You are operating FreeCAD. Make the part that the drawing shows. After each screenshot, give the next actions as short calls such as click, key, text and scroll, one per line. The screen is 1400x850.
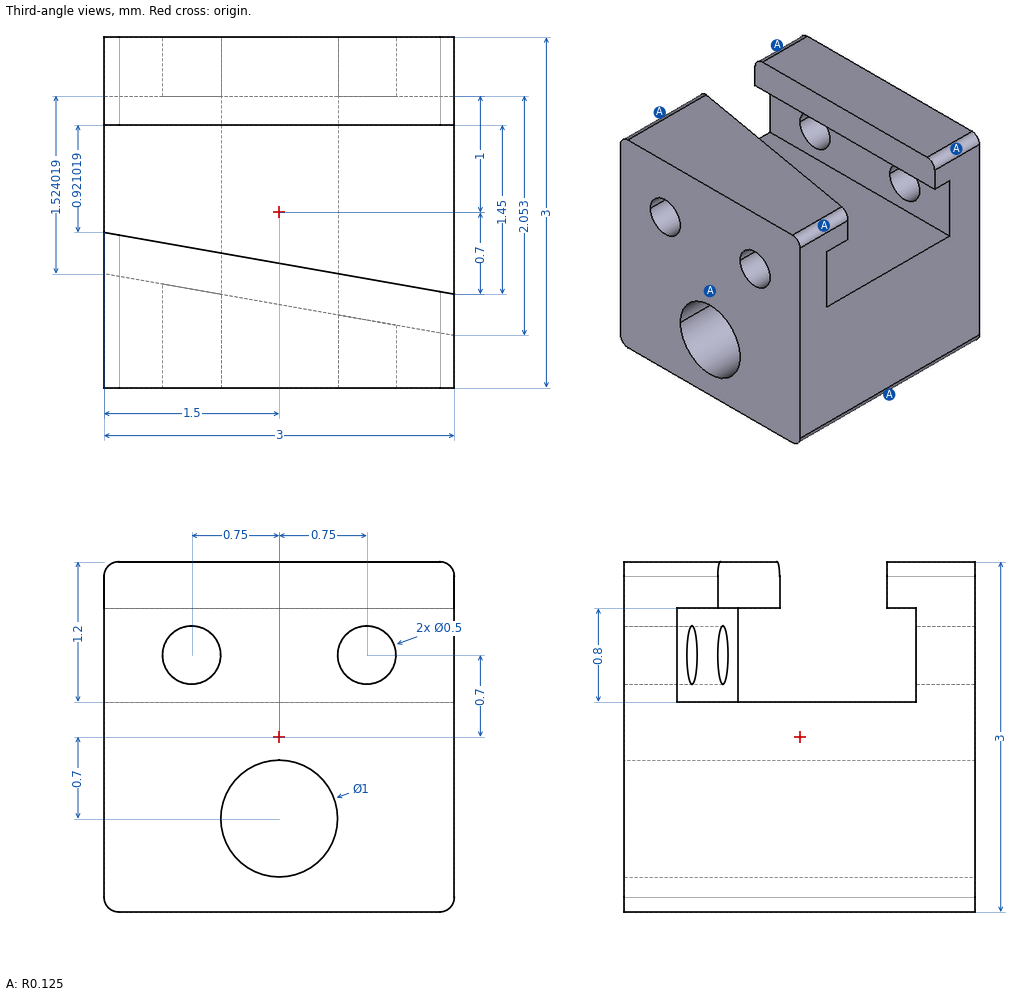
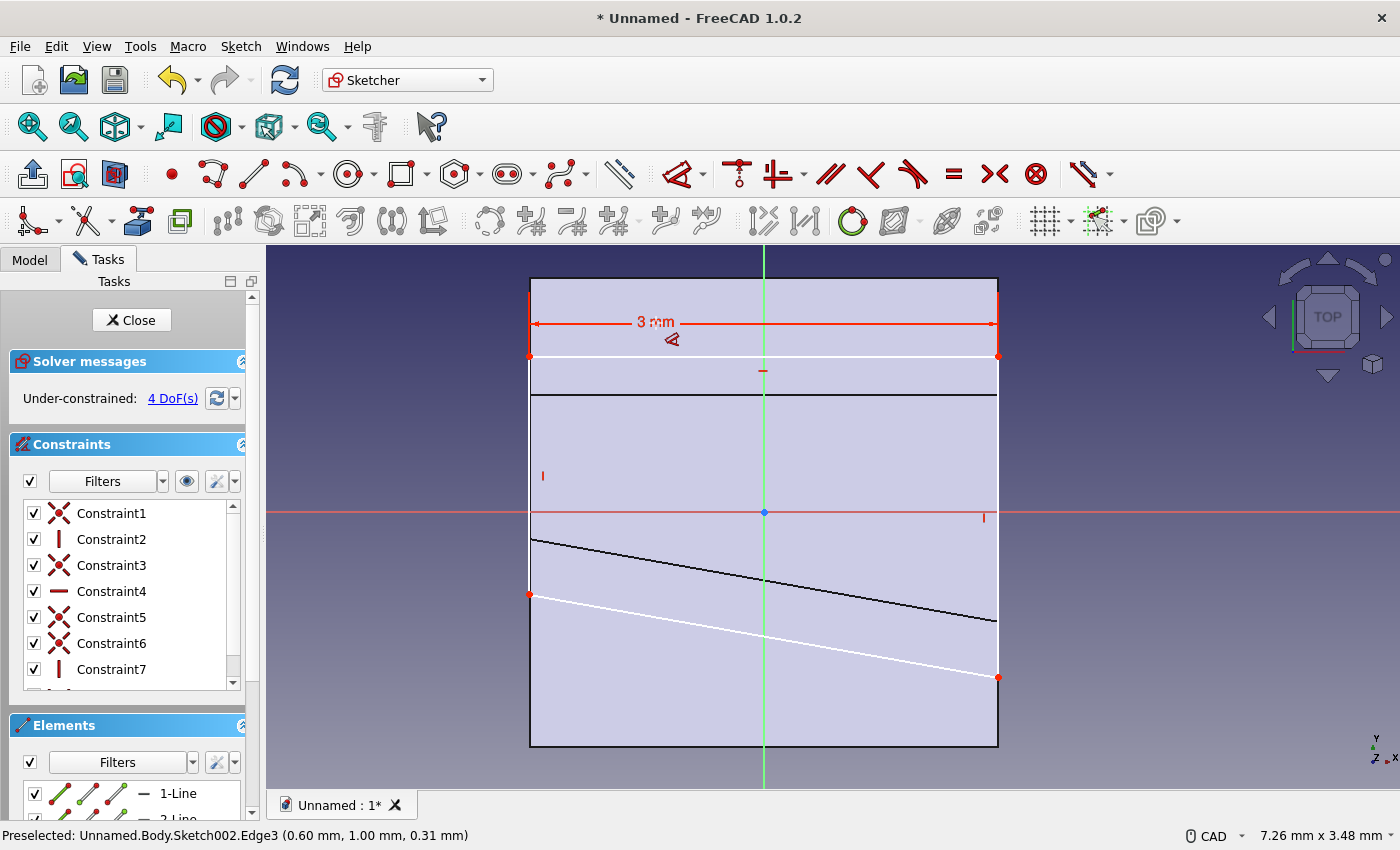
click(998, 357)
click(1032, 435)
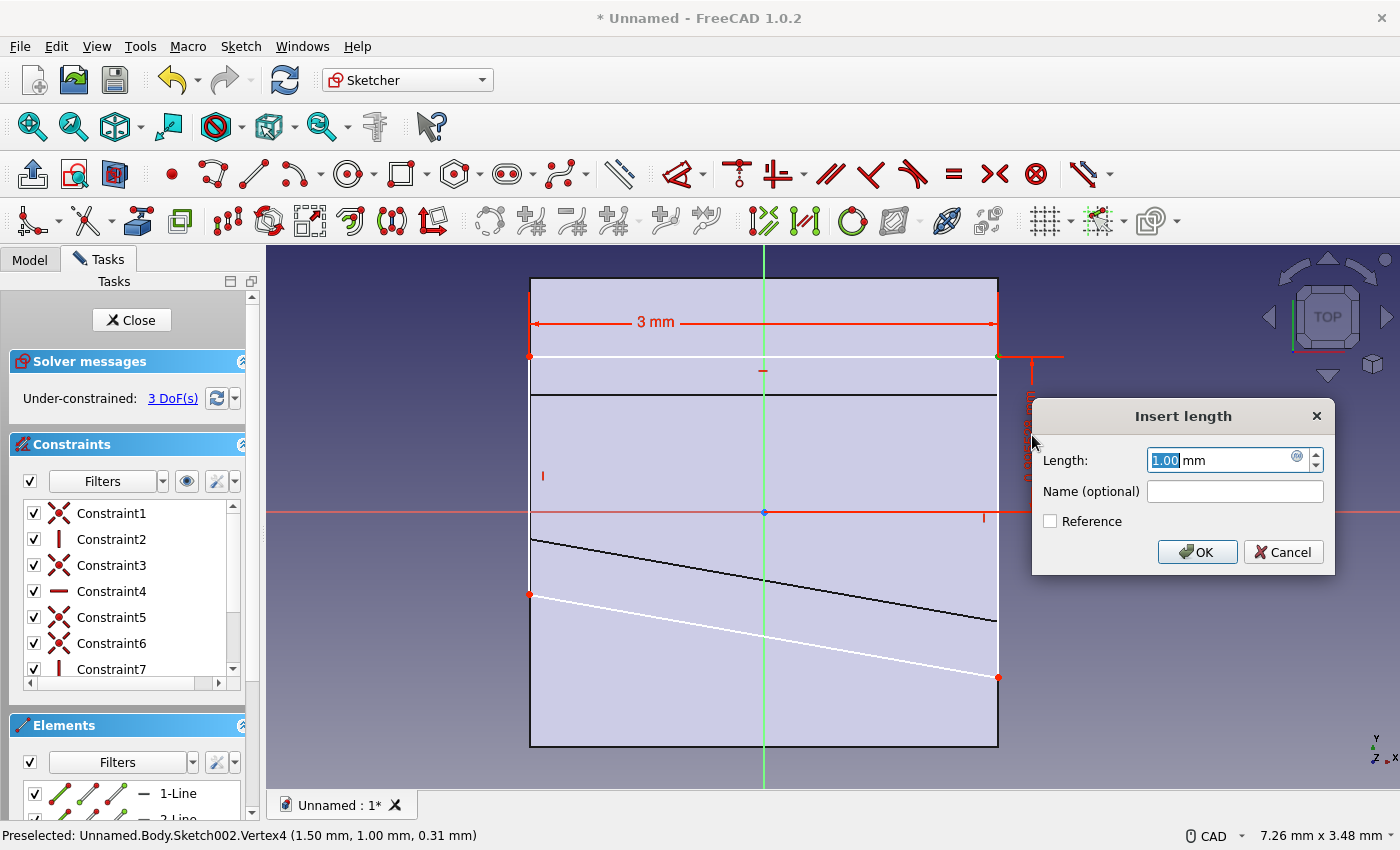
text(1)
key(Return)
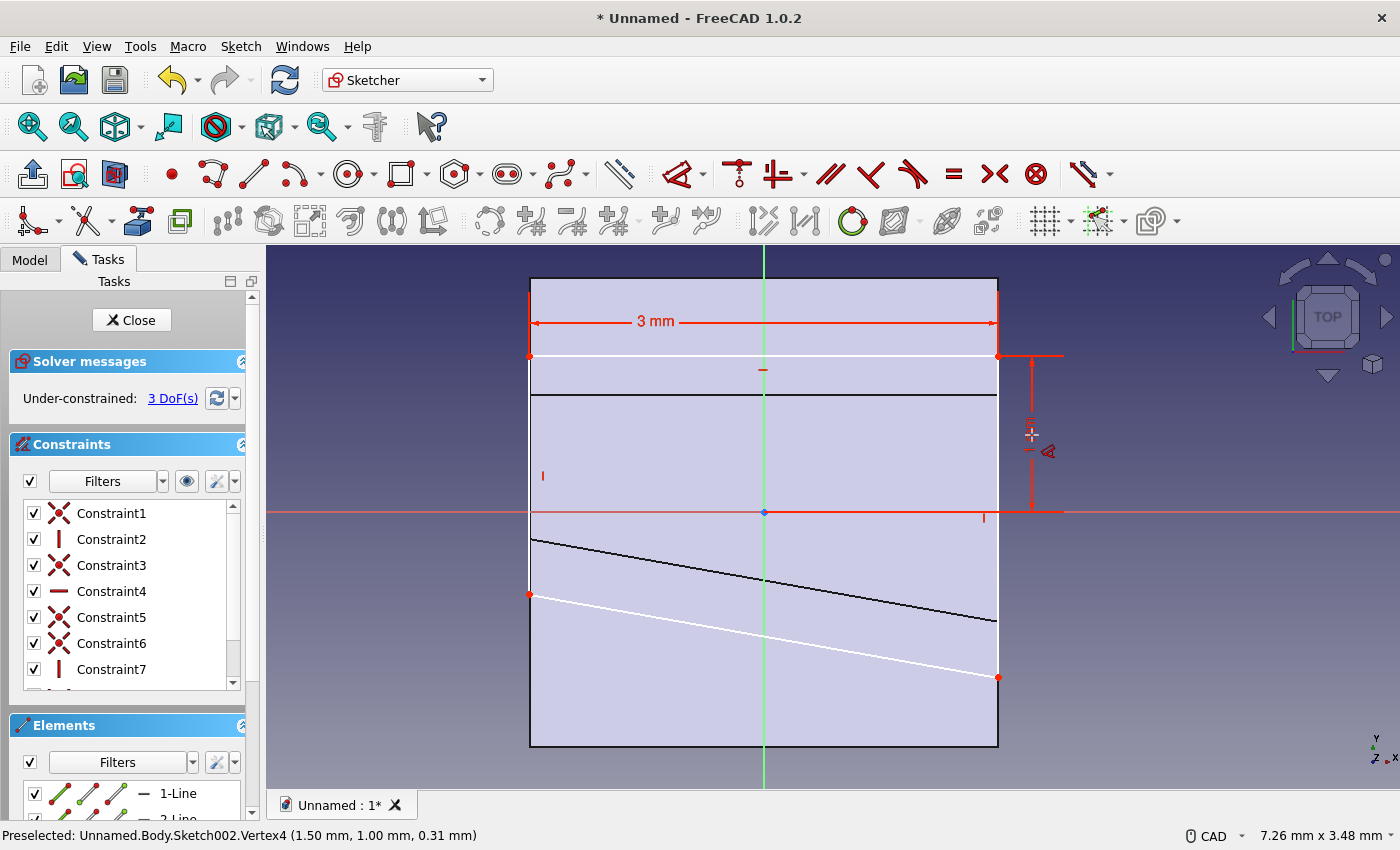
click(529, 595)
click(647, 629)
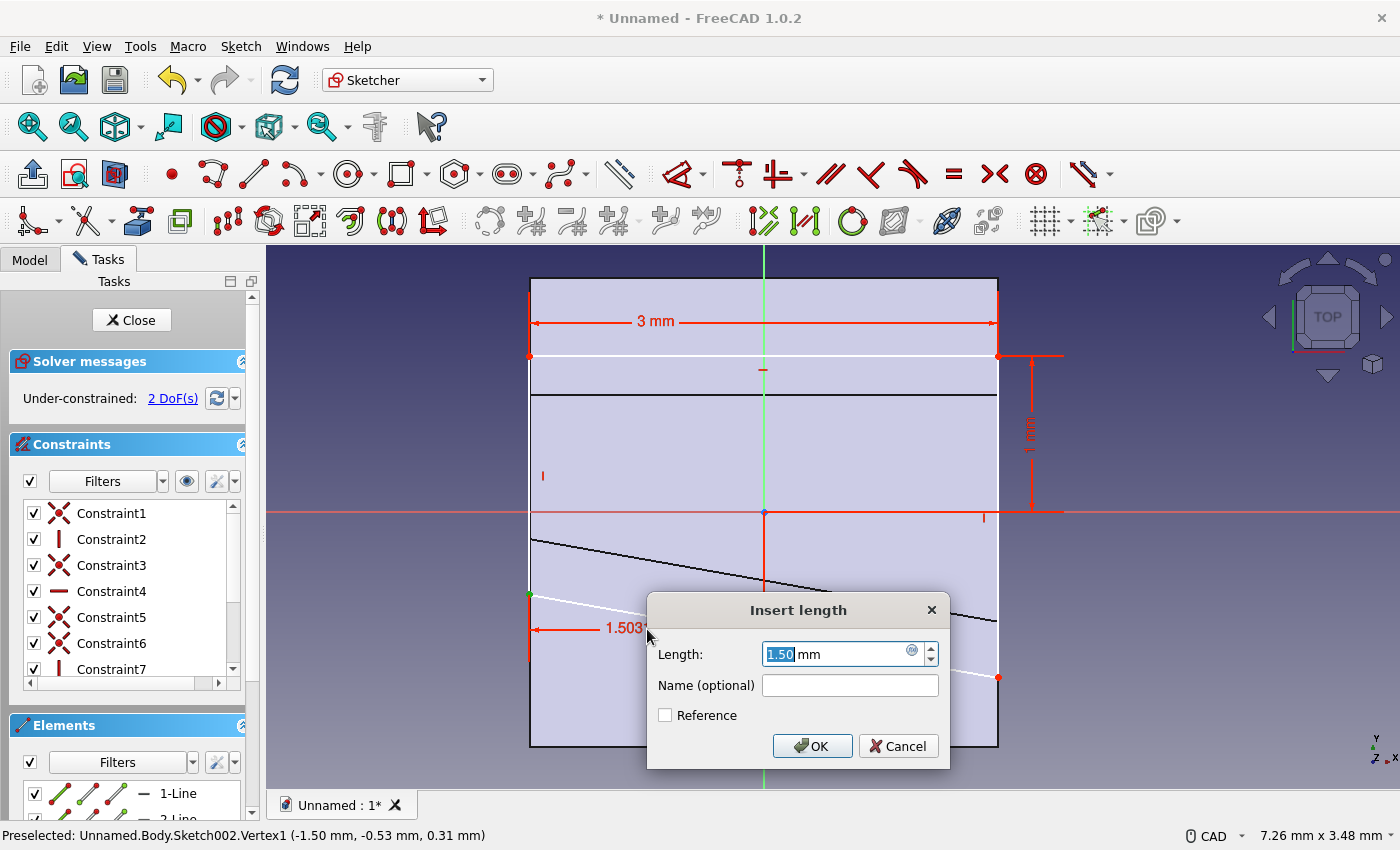
text(1.5)
key(Return)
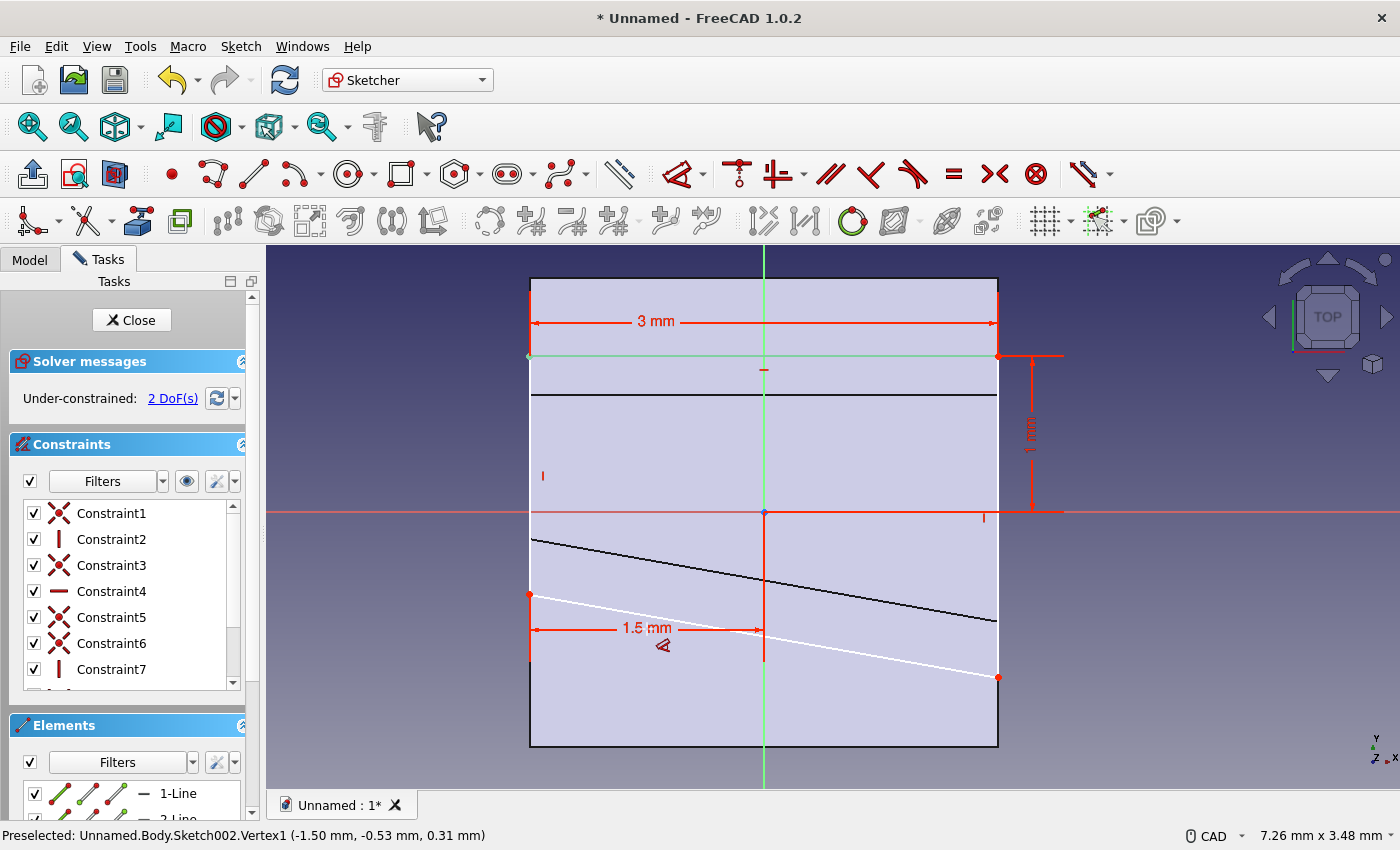
click(998, 581)
click(1032, 591)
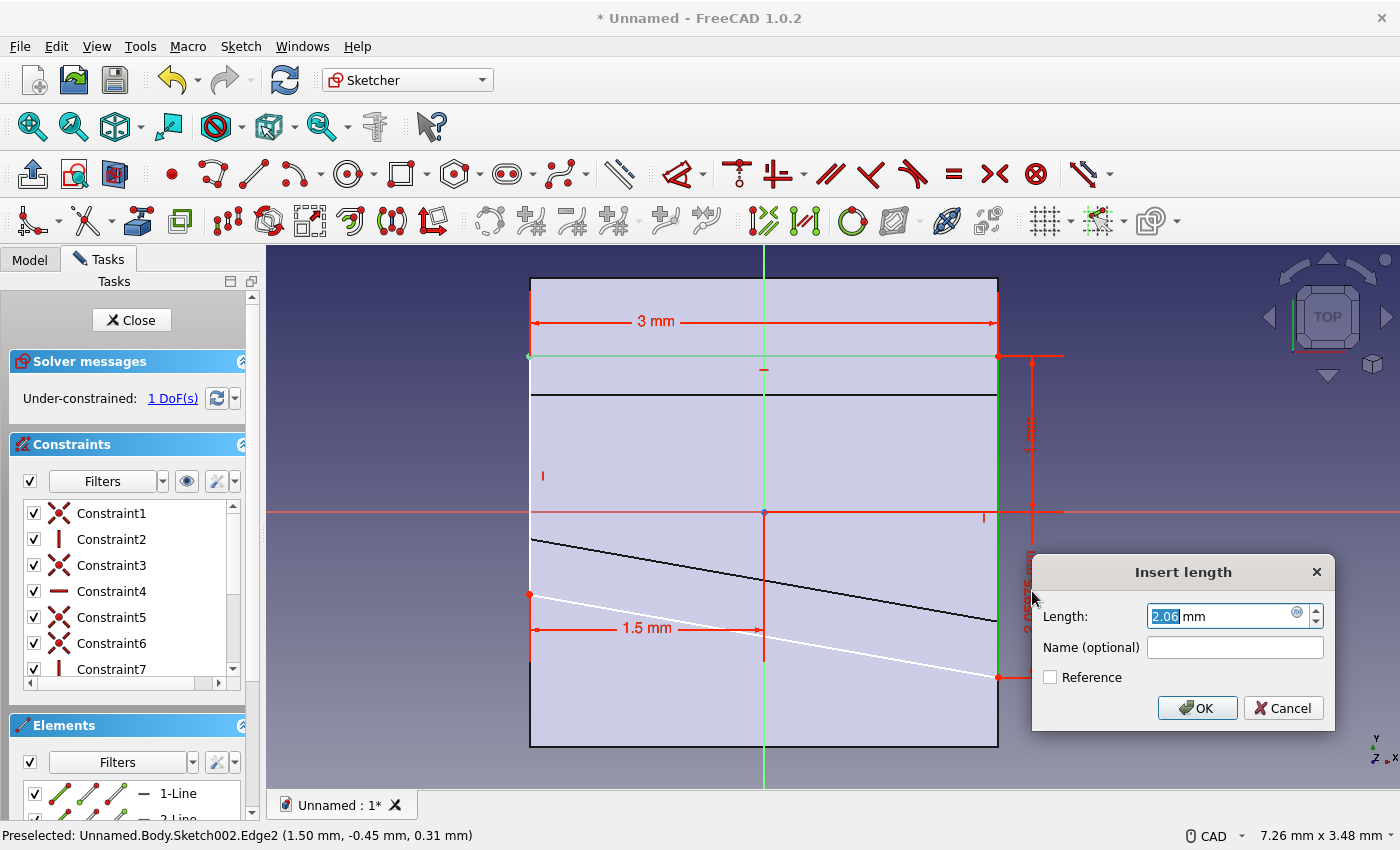
text(2.053)
key(Return)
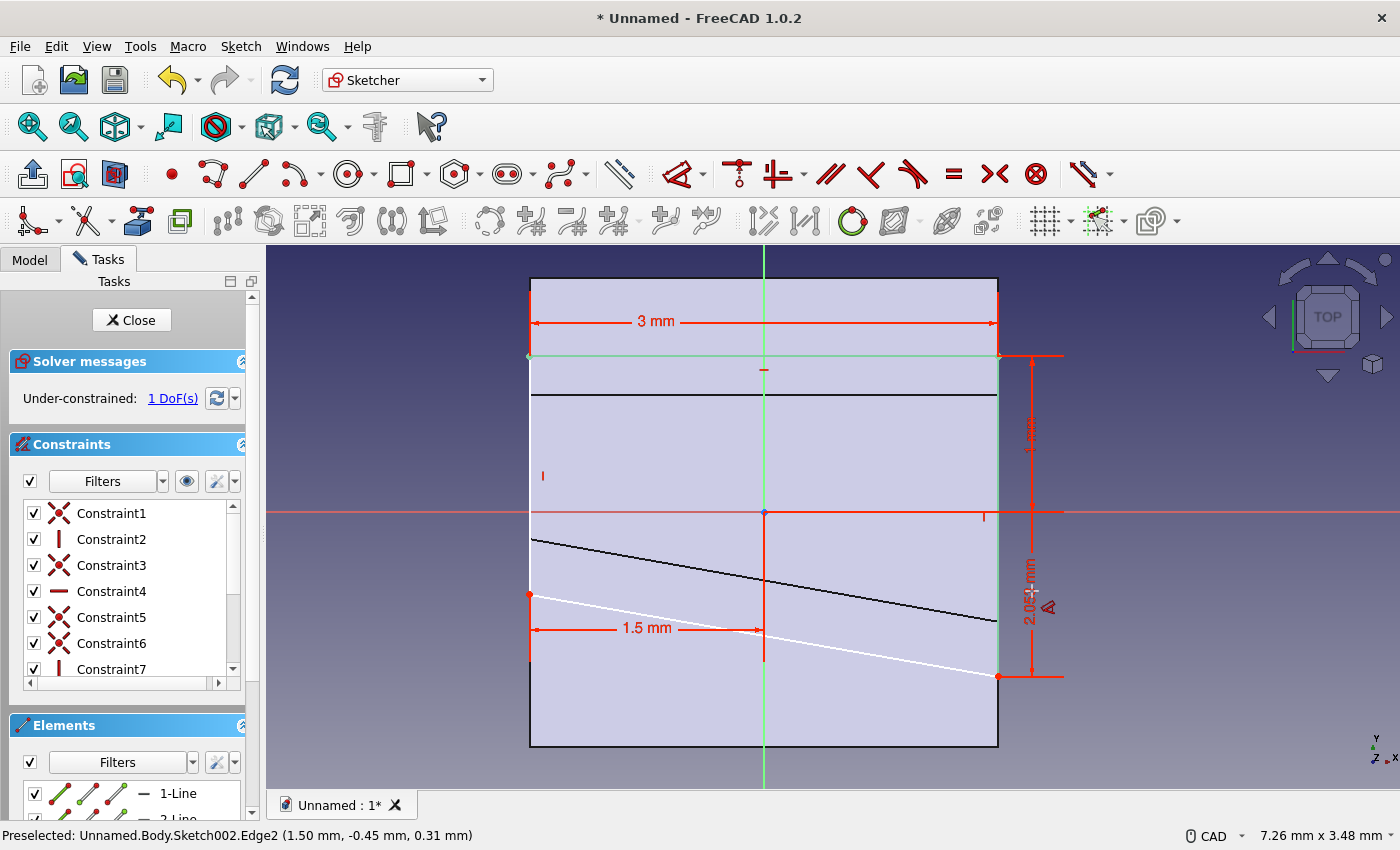
click(530, 428)
click(496, 476)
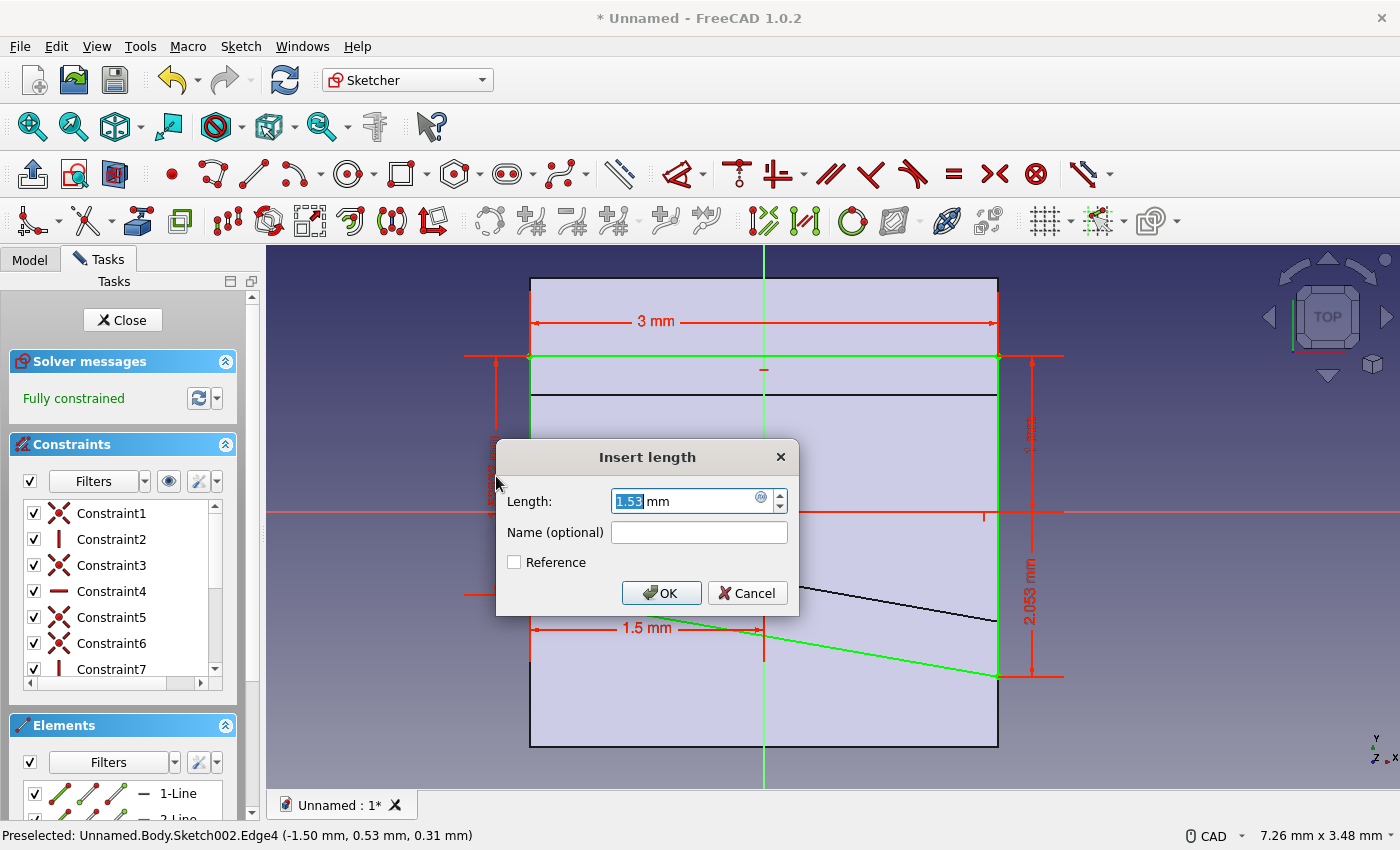
text(1.524019)
key(Return)
key(Escape)